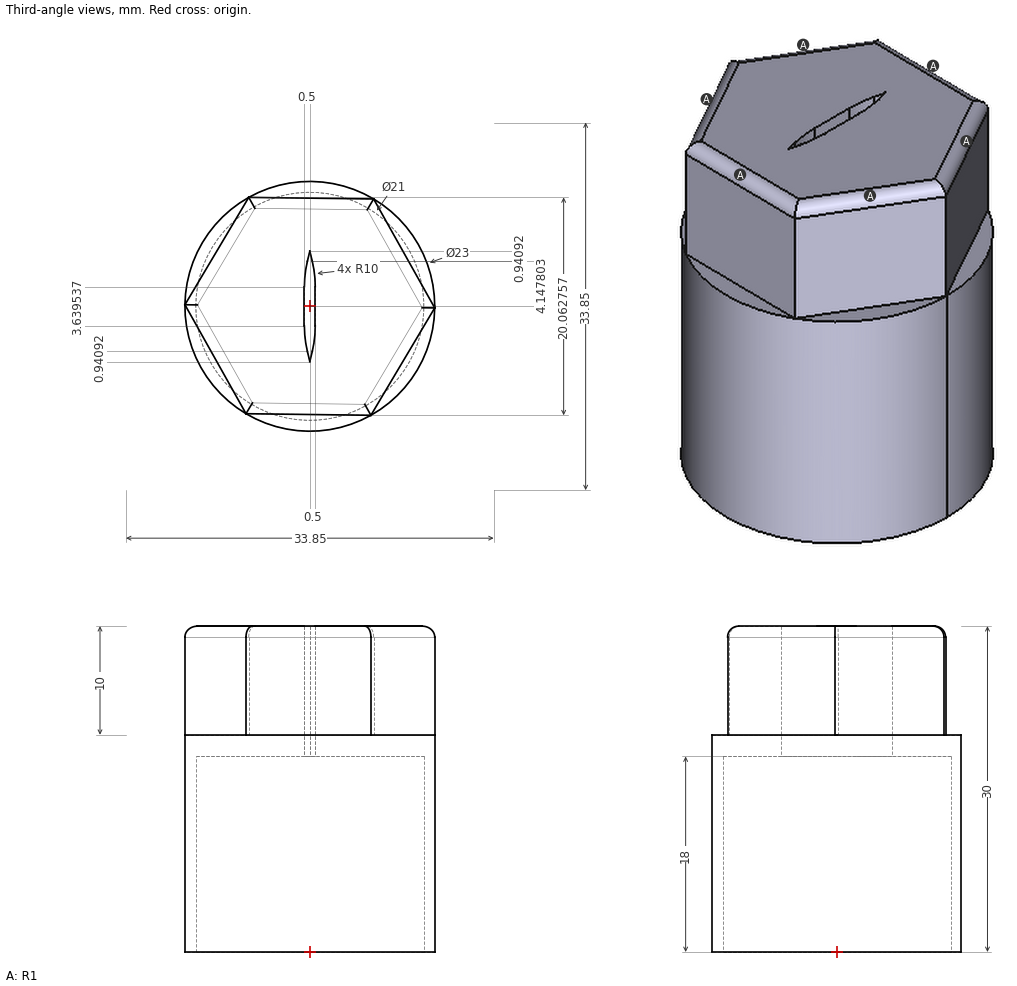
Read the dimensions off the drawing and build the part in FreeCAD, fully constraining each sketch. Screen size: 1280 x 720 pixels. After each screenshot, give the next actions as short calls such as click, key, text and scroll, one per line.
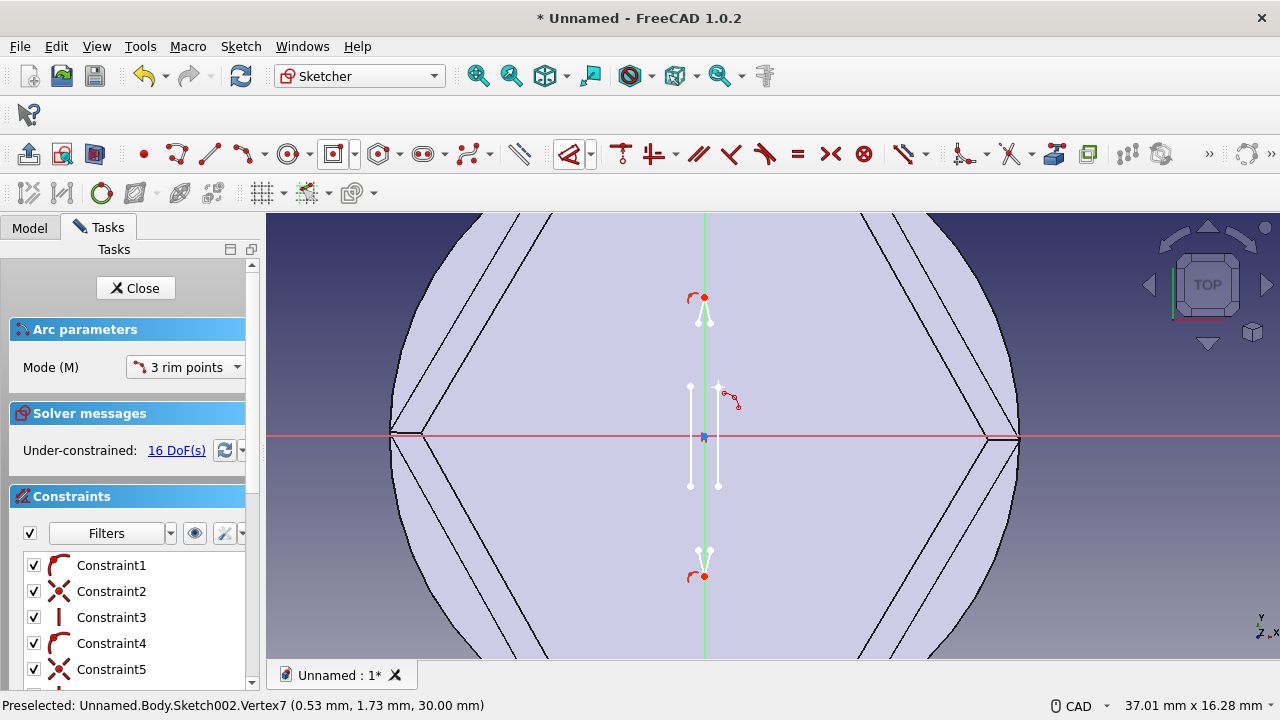
scroll(698, 323, up, 5)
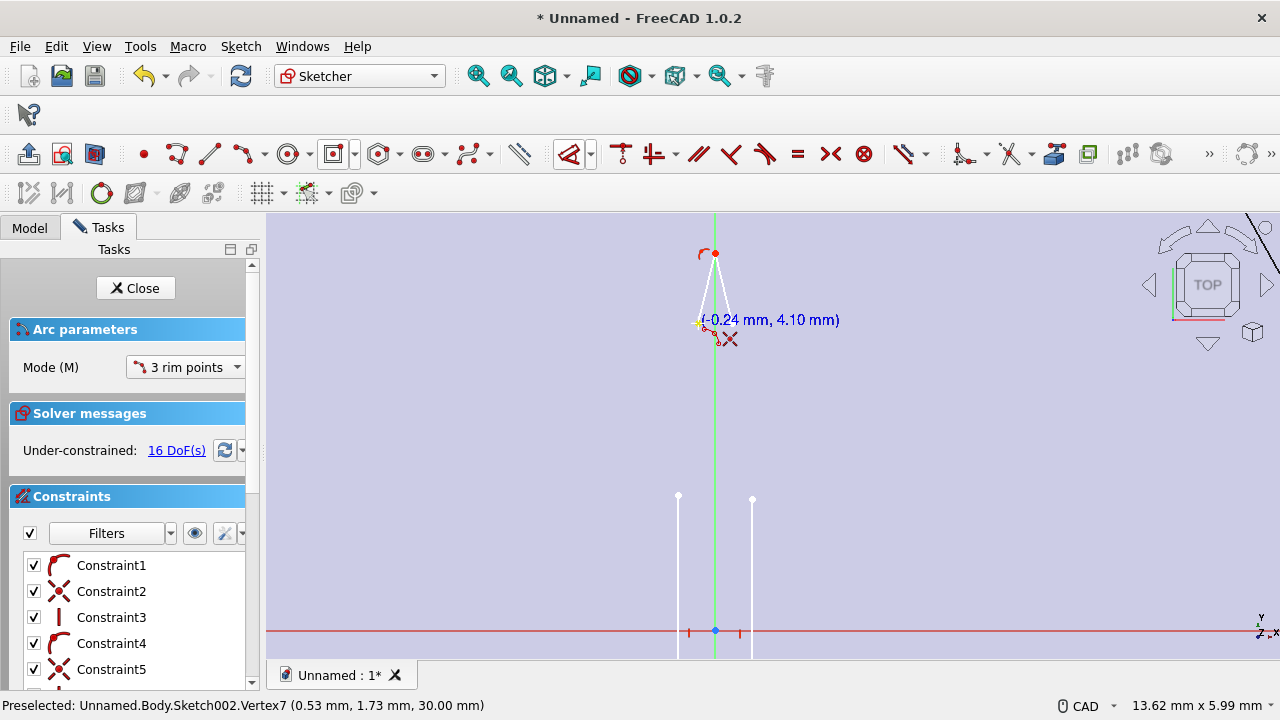
click(698, 323)
click(678, 496)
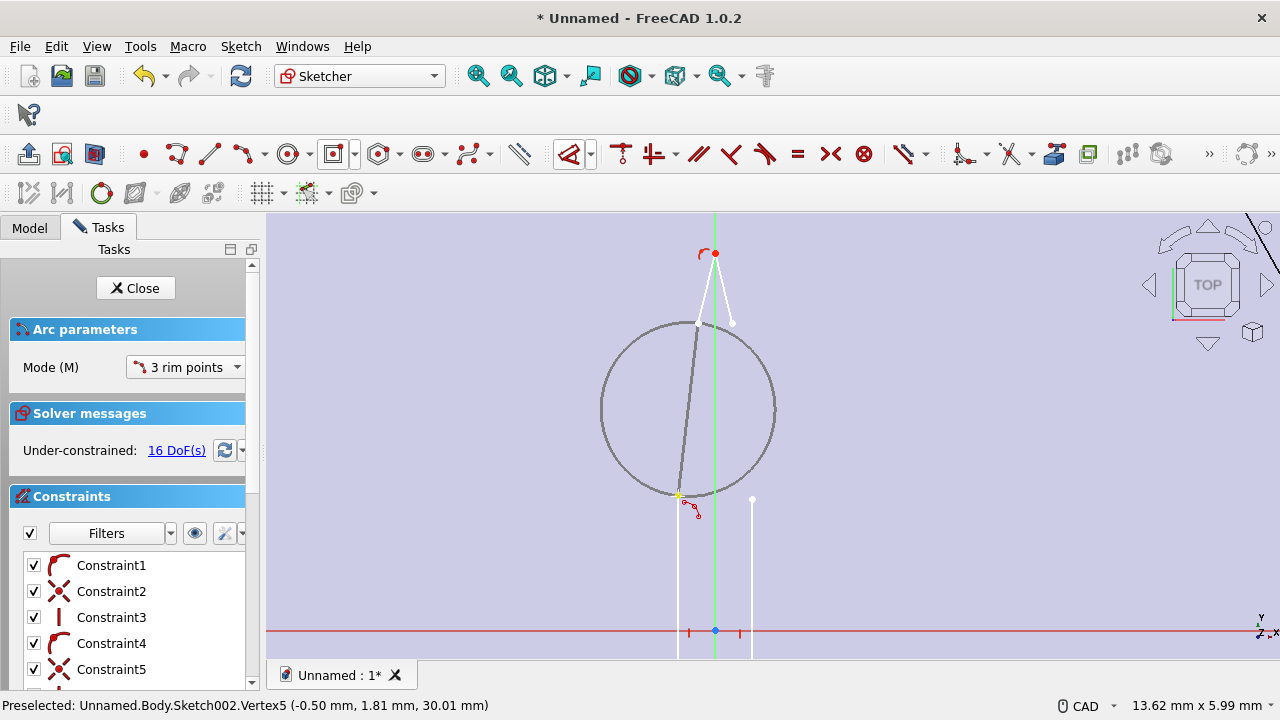
scroll(683, 408, up, 6)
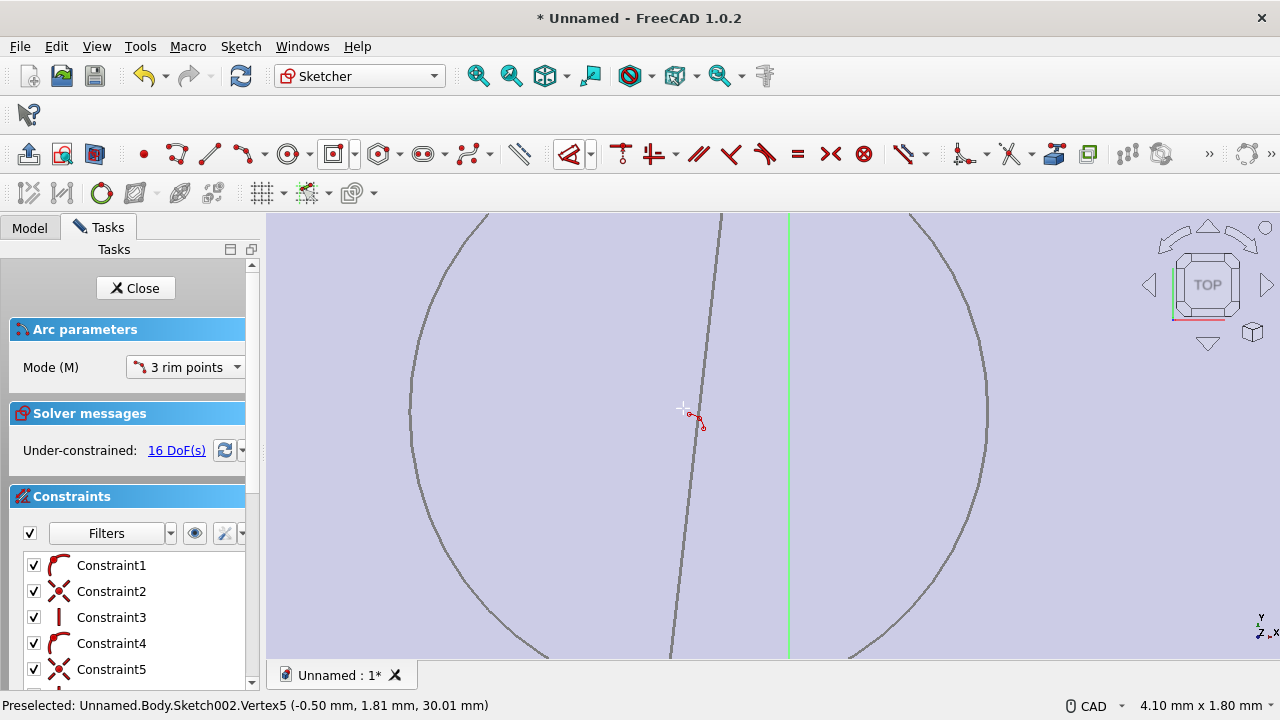
click(682, 407)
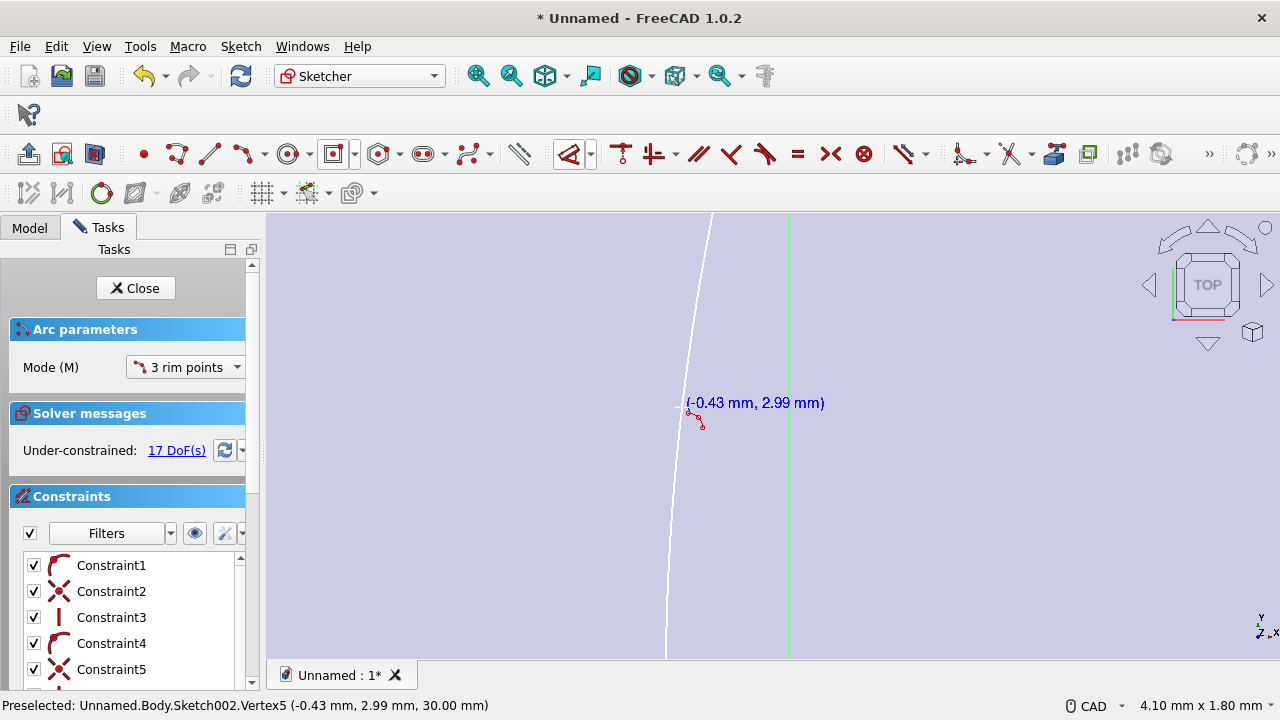
scroll(694, 347, down, 11)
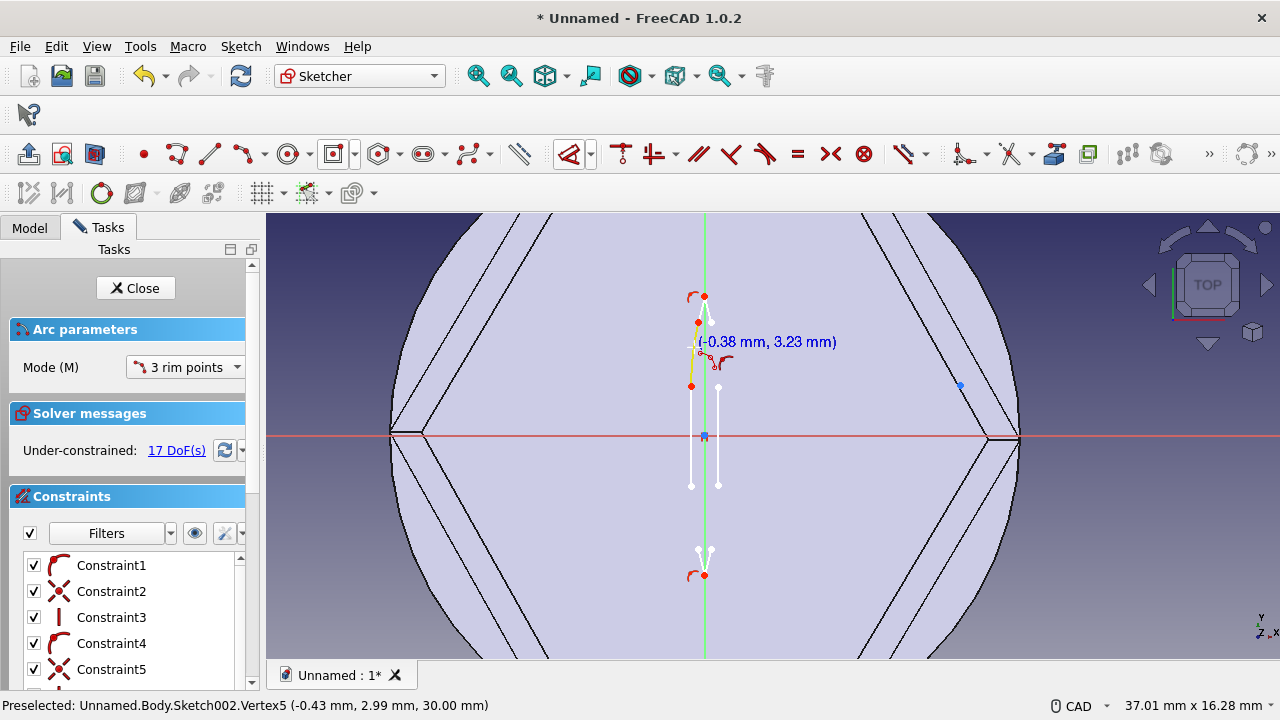
click(691, 486)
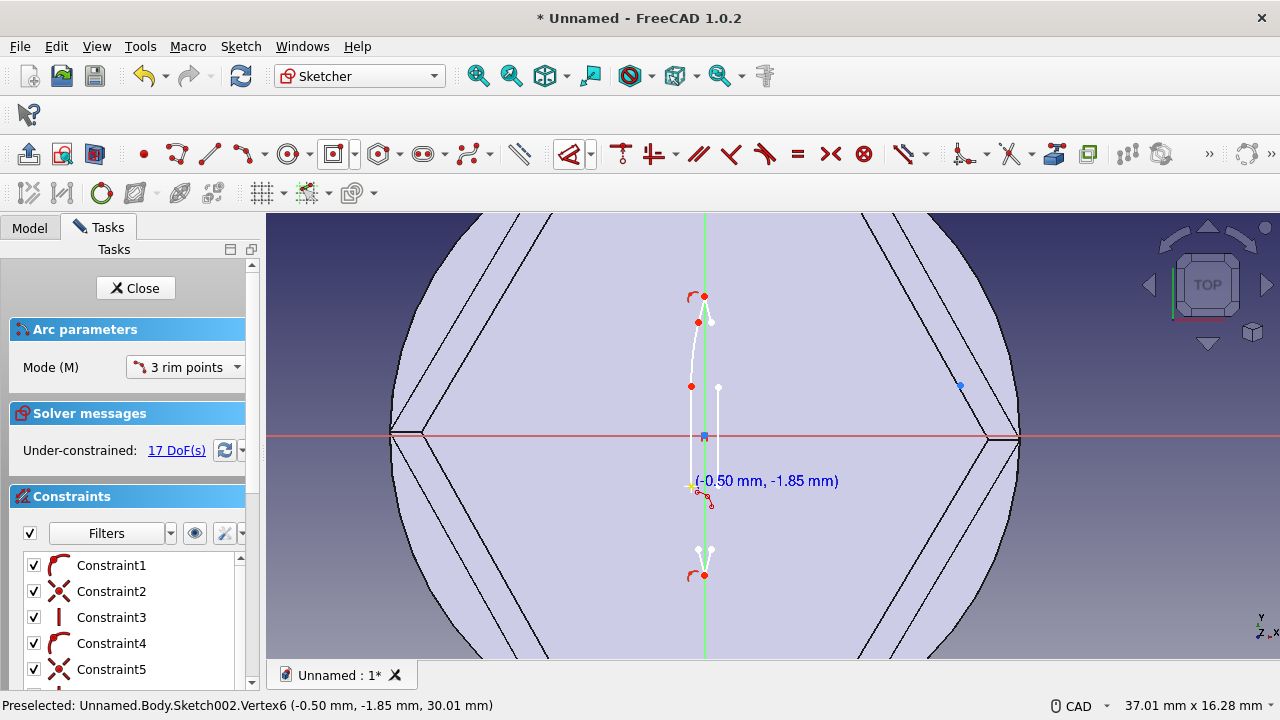
scroll(699, 550, up, 5)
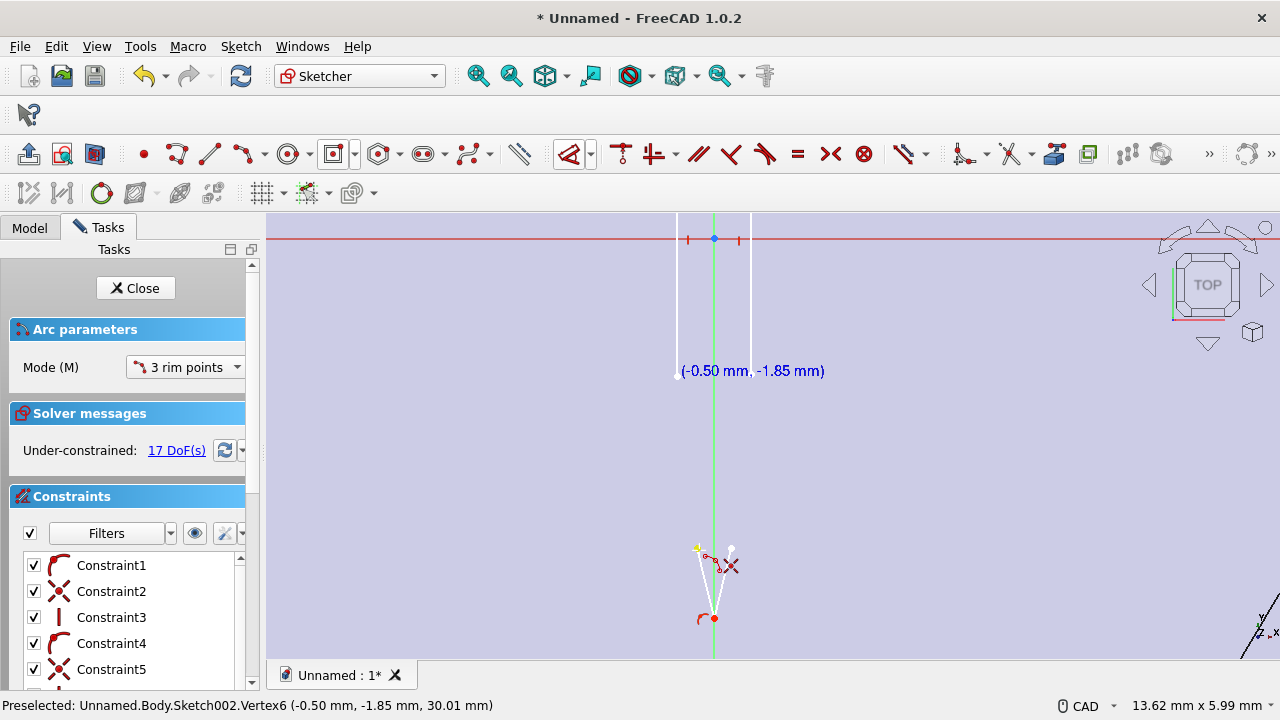
click(697, 549)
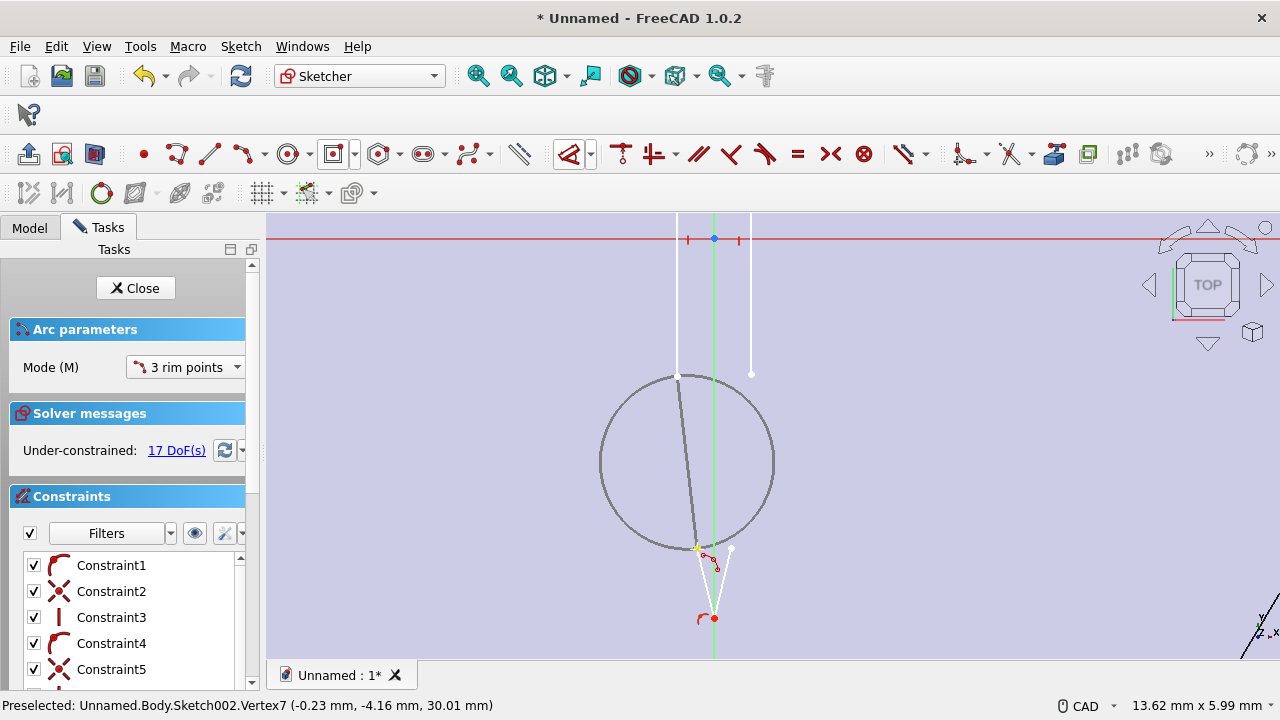
scroll(682, 461, up, 6)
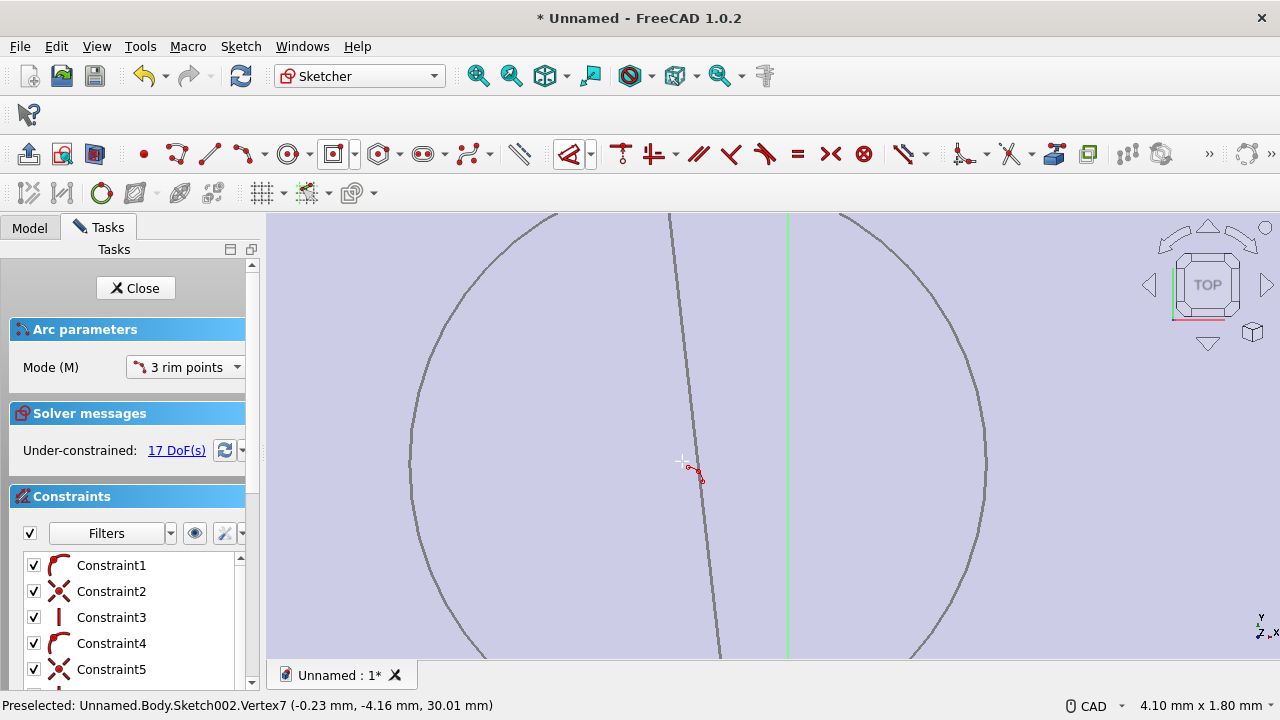
click(682, 461)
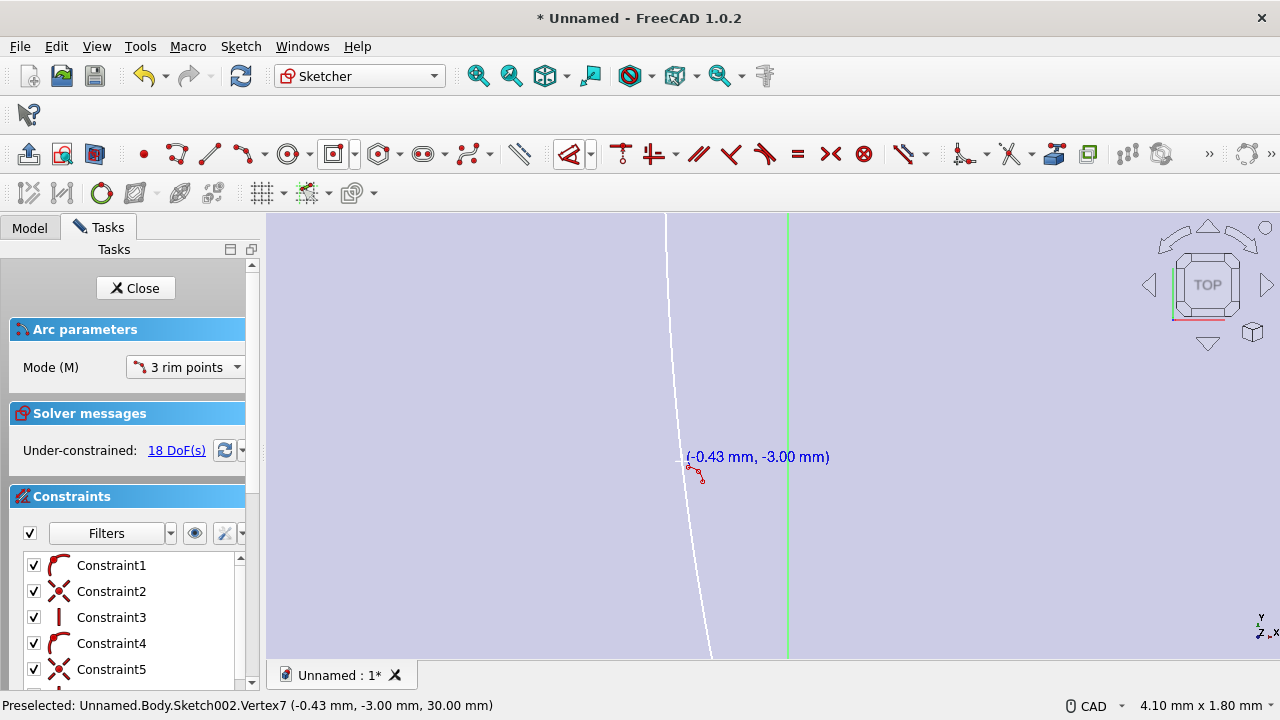
scroll(694, 525, down, 11)